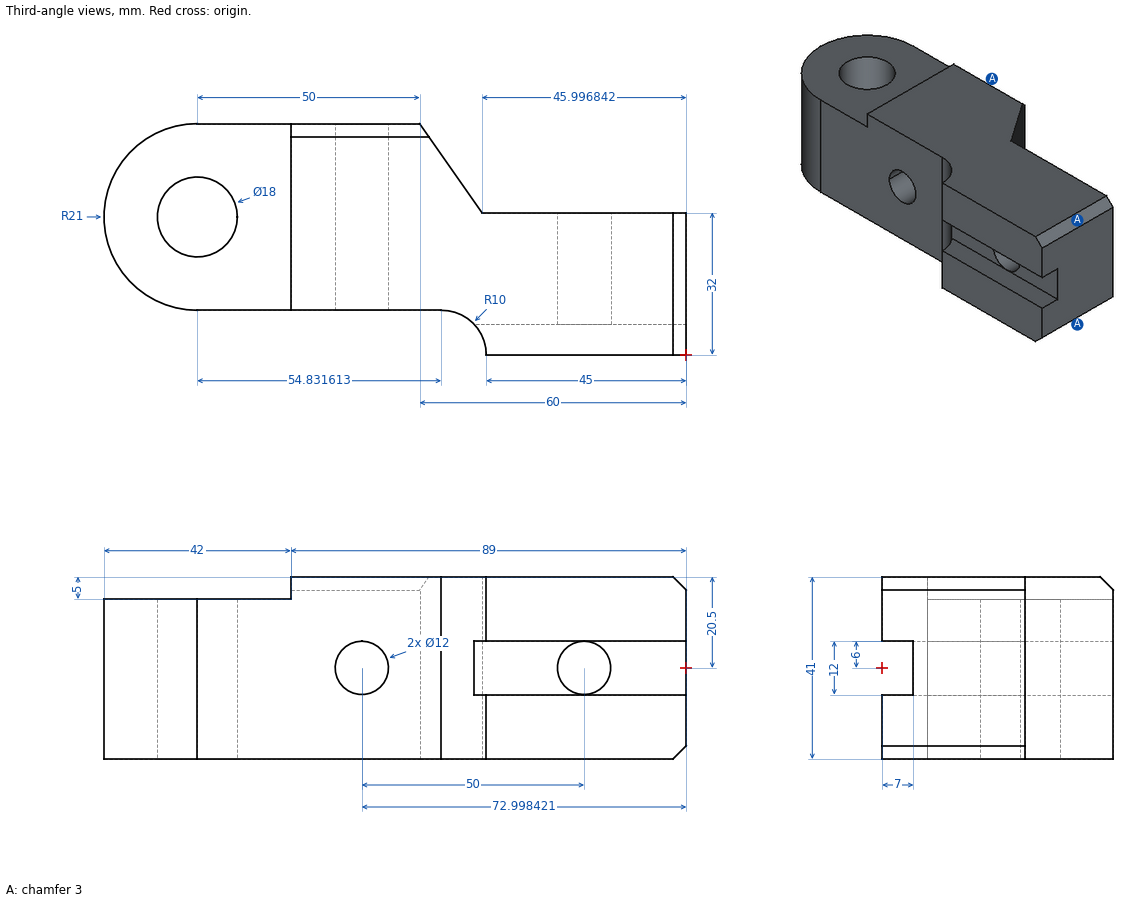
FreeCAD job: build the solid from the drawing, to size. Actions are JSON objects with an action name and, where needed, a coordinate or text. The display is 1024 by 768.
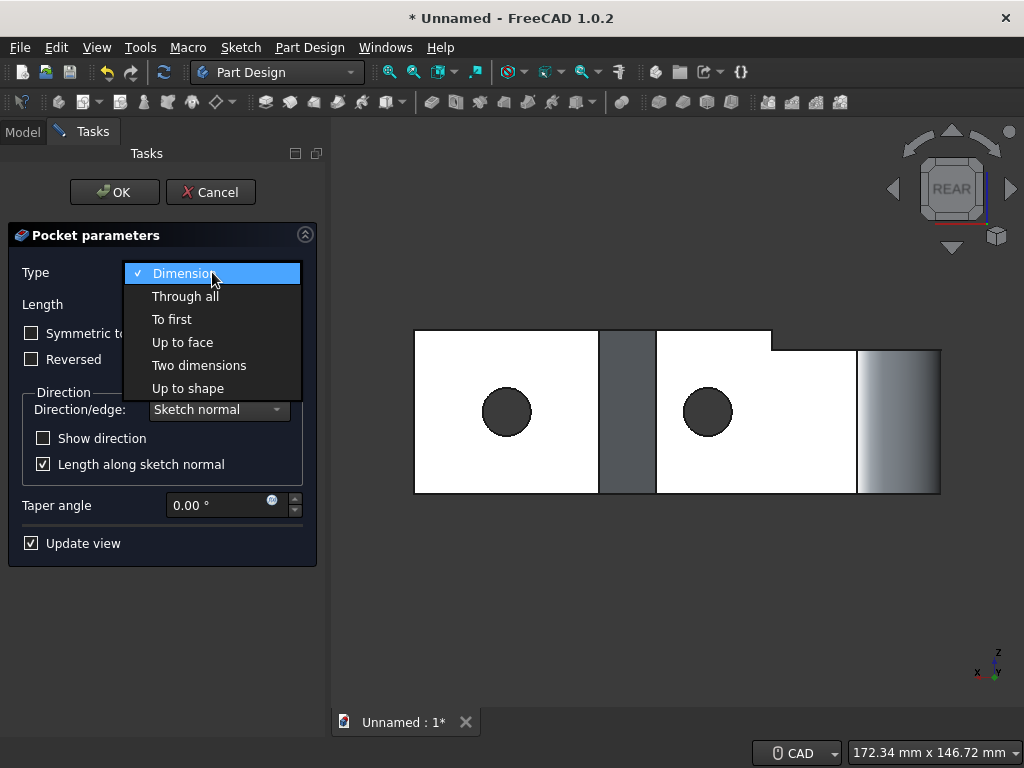
{"action": "left_click", "coordinate": [212, 296]}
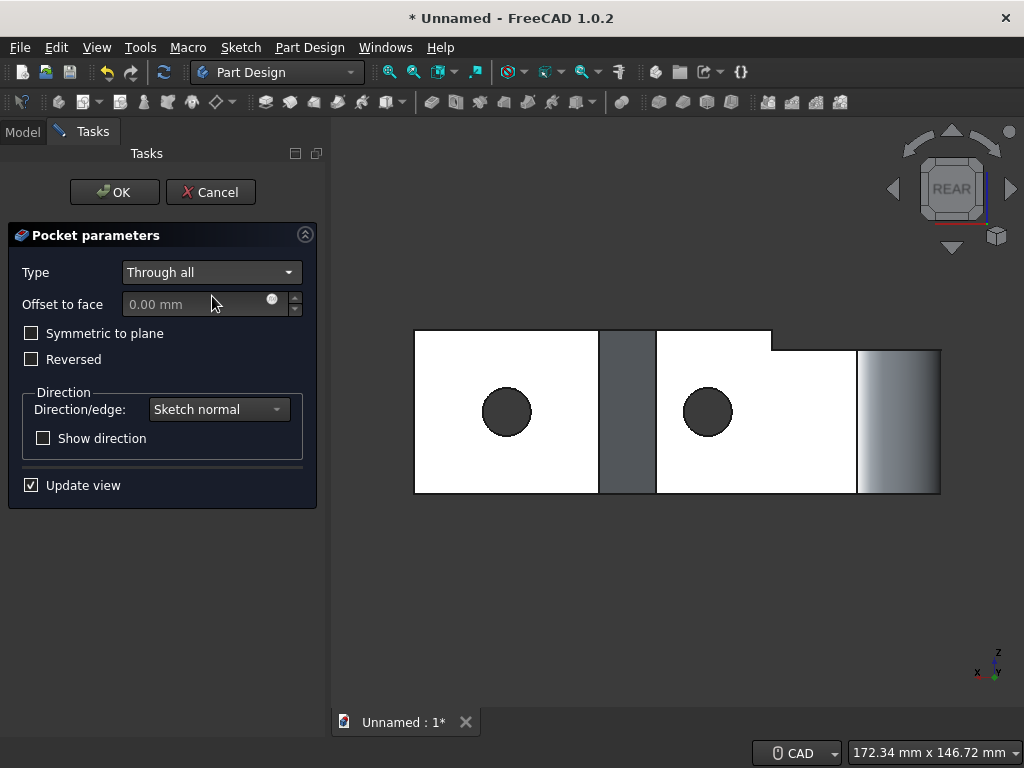
{"action": "left_click", "coordinate": [115, 192]}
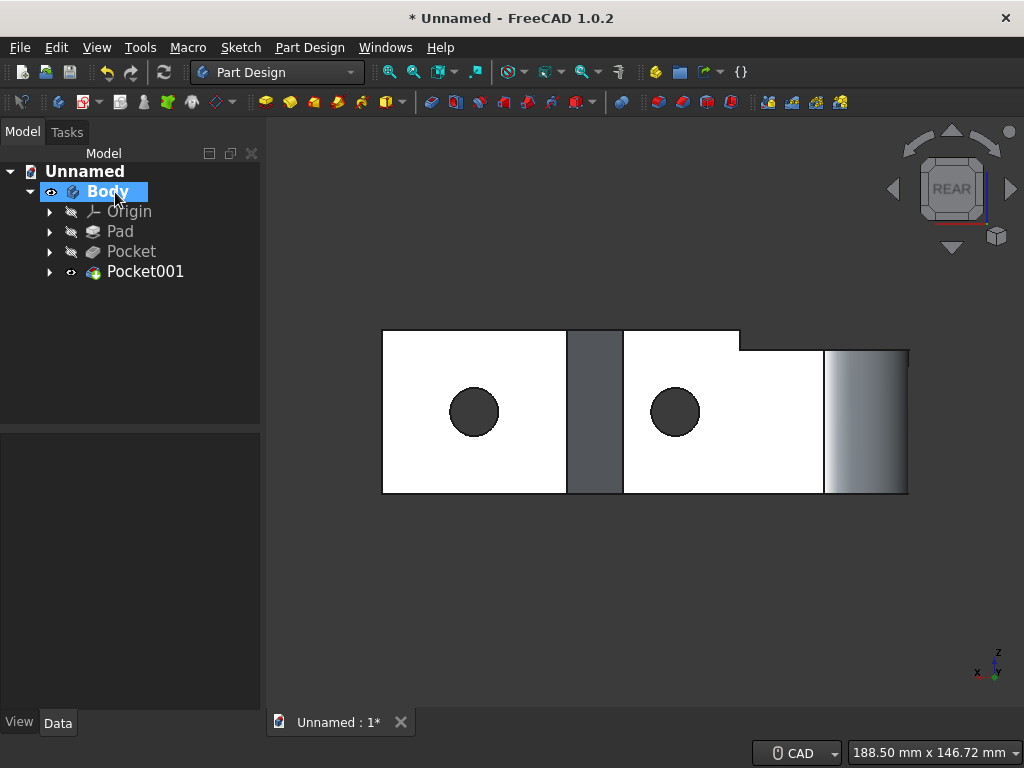
{"action": "left_click", "coordinate": [681, 329]}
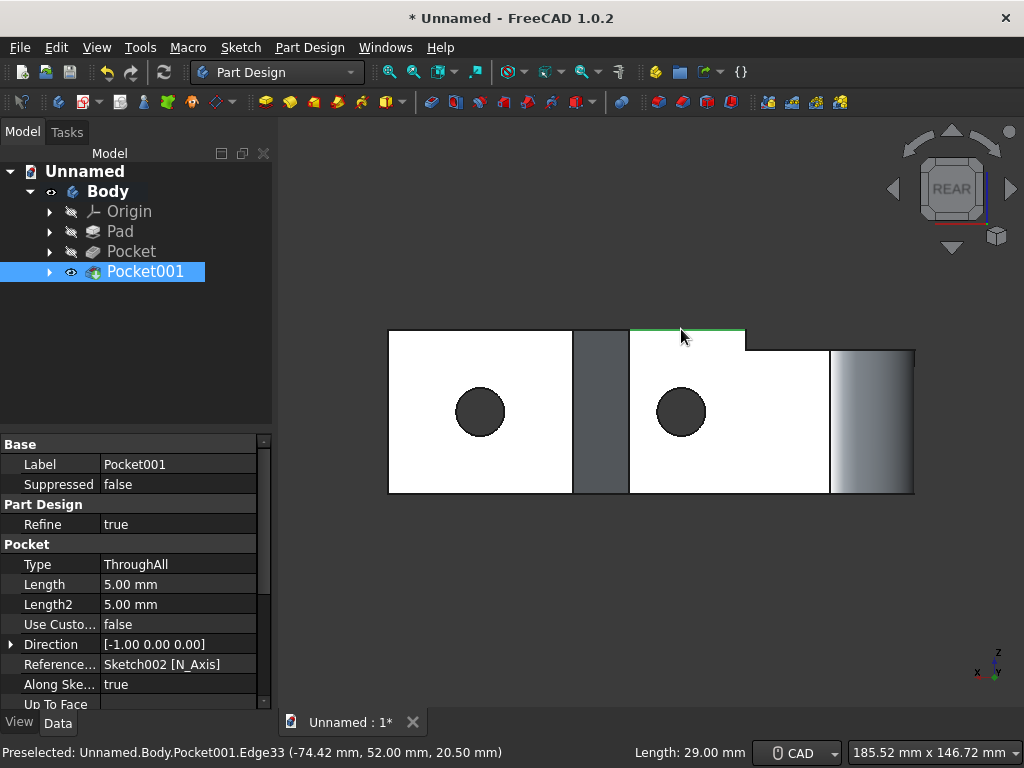
{"action": "key", "text": "0"}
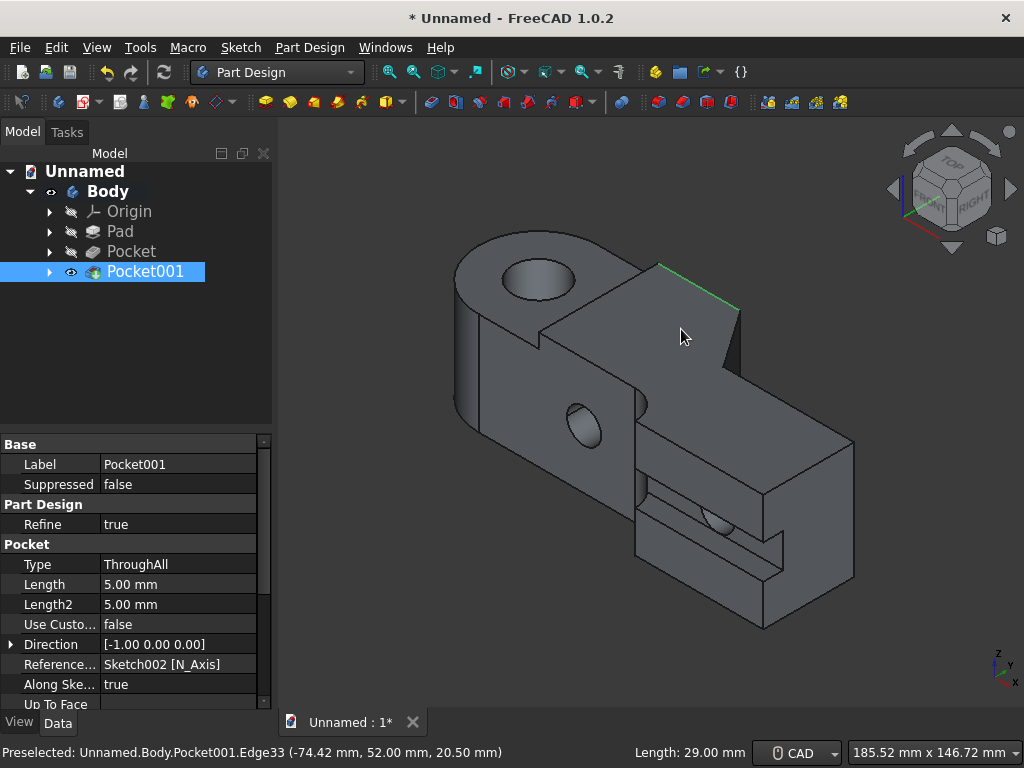
{"action": "left_click", "coordinate": [809, 468], "text": "ctrl"}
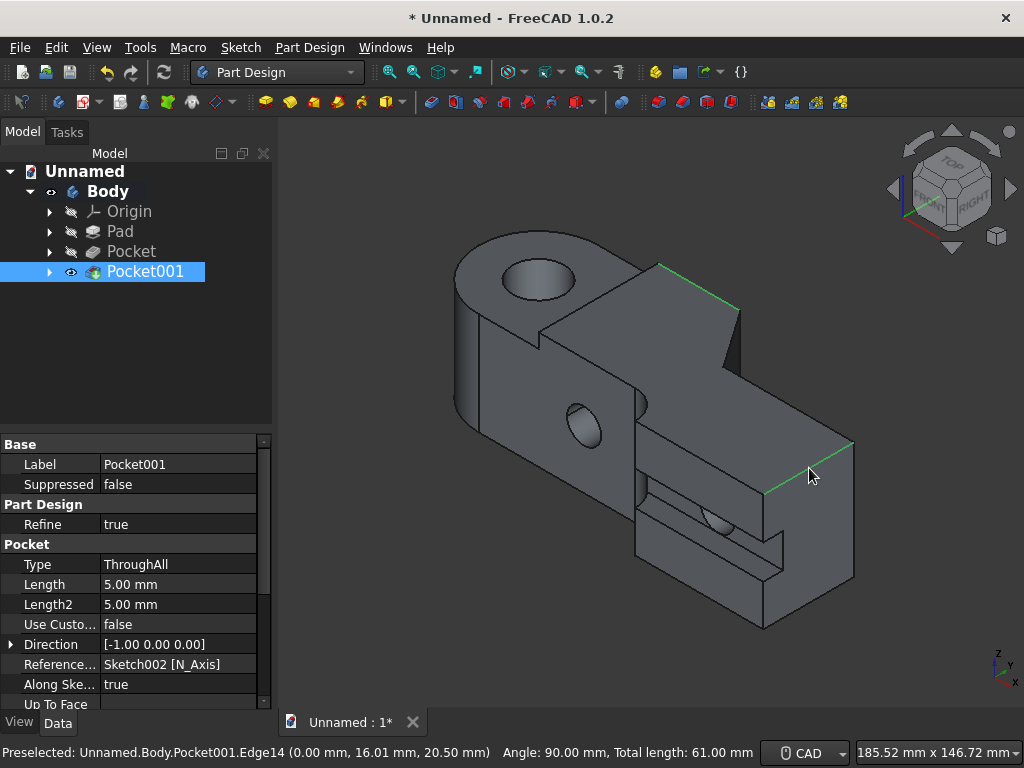
{"action": "key", "text": "2"}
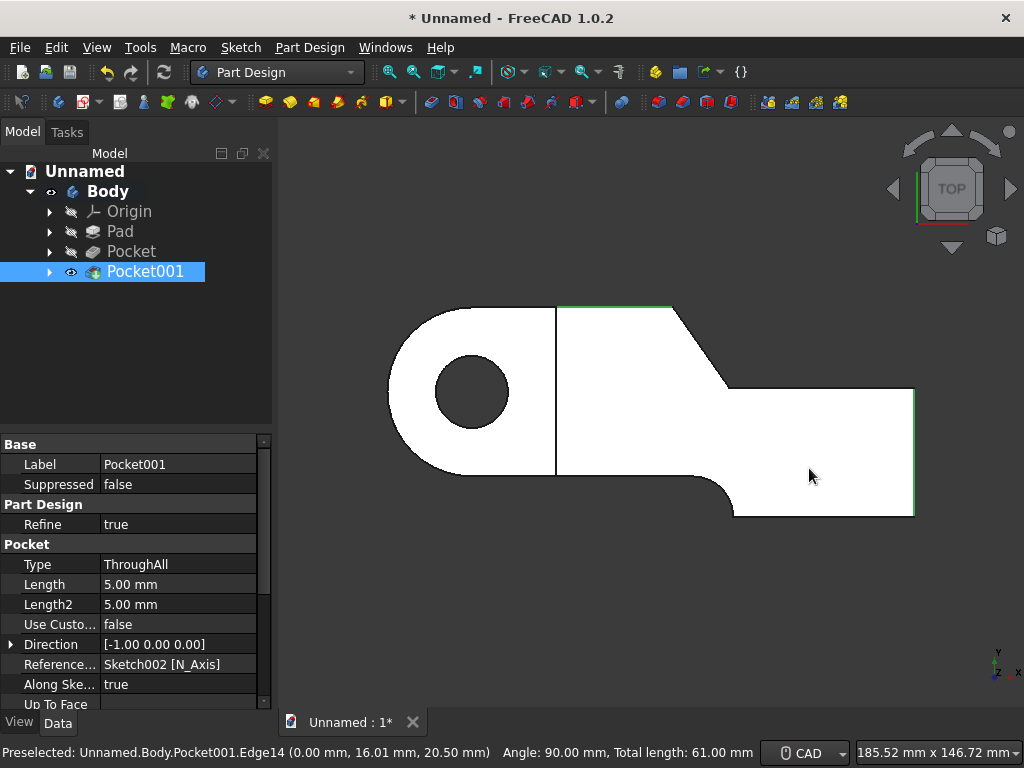
{"action": "key", "text": "1"}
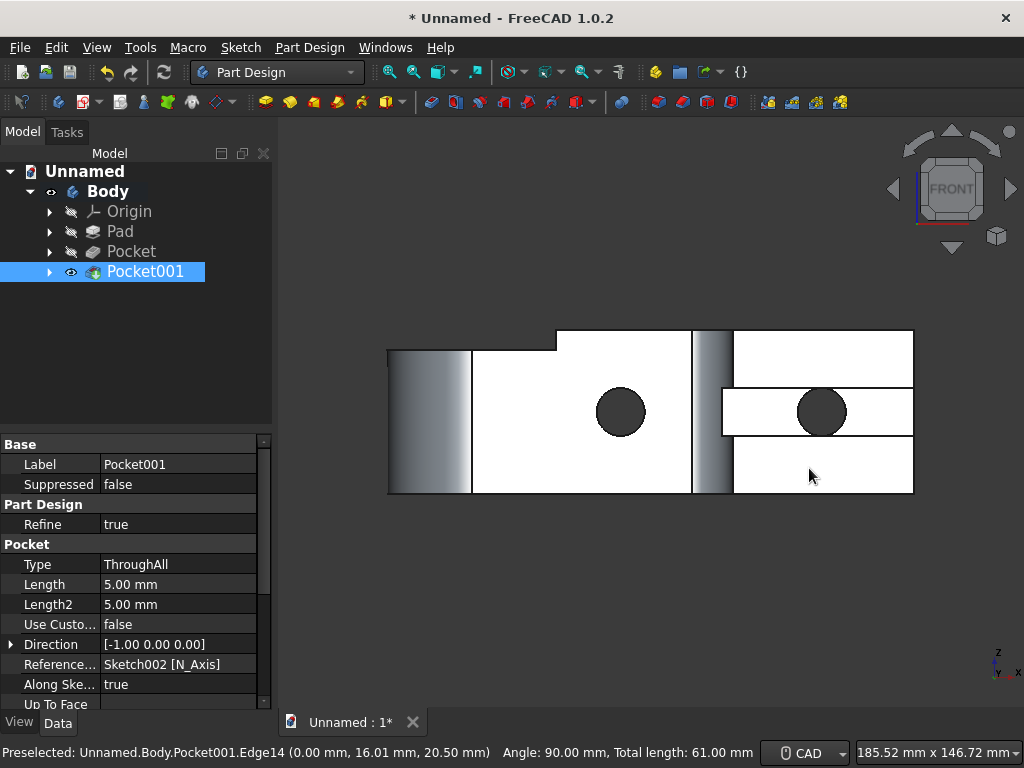
{"action": "key", "text": "3"}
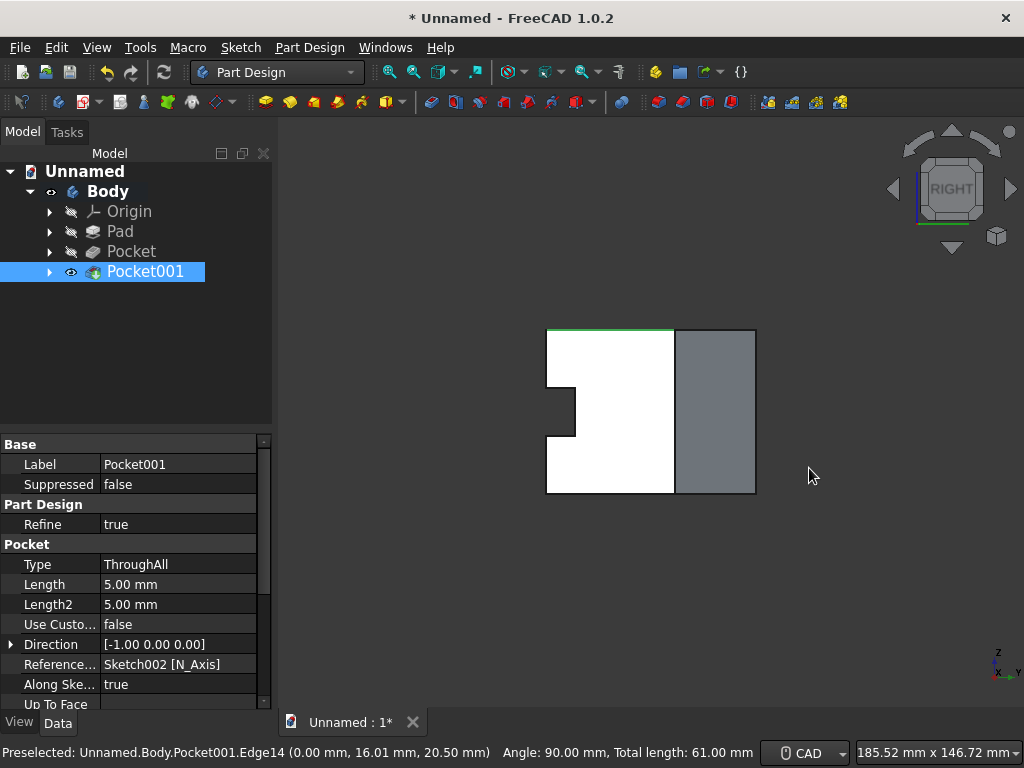
{"action": "left_click", "coordinate": [390, 72]}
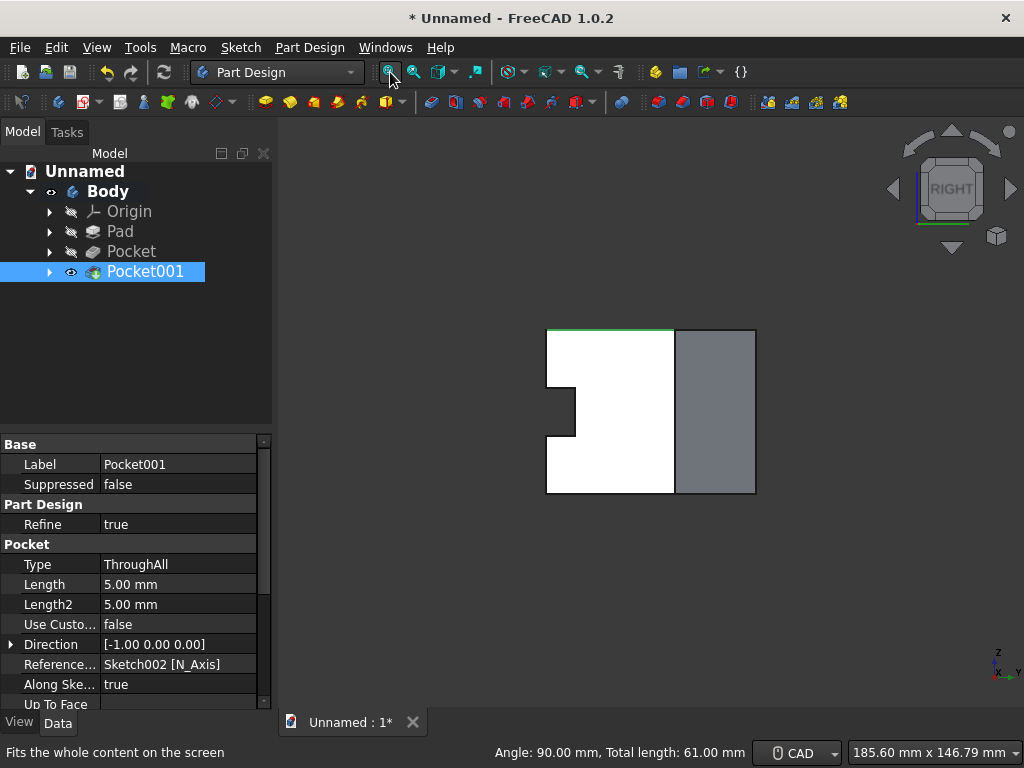
{"action": "left_click", "coordinate": [611, 493], "text": "ctrl"}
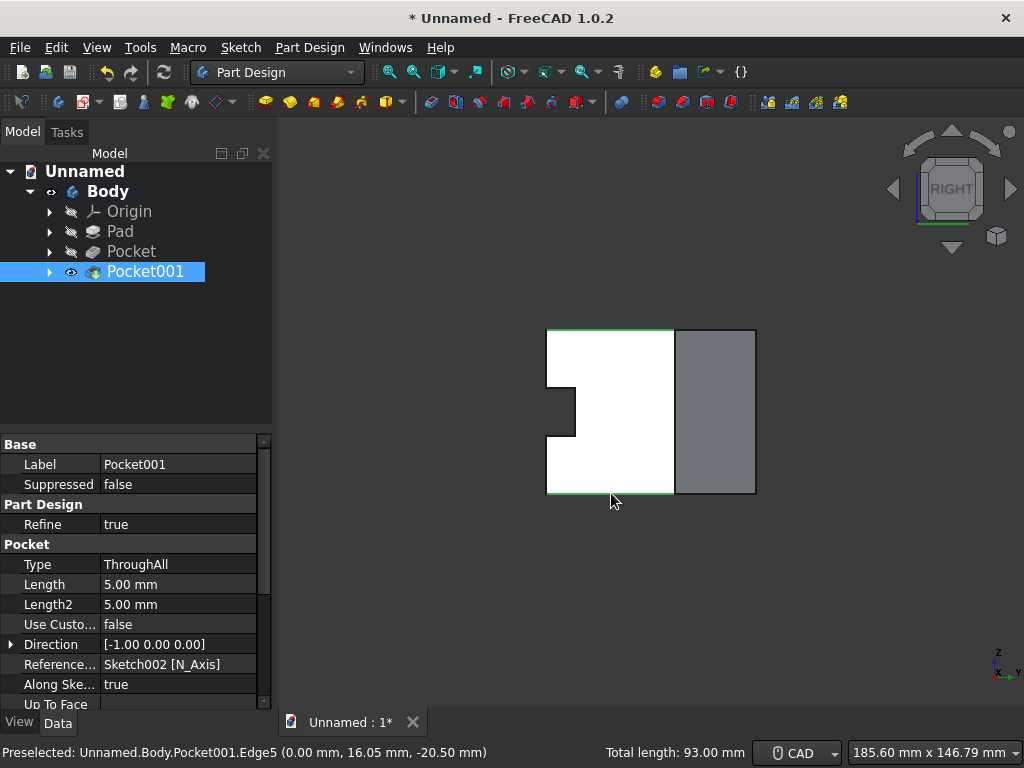
{"action": "left_click", "coordinate": [684, 102]}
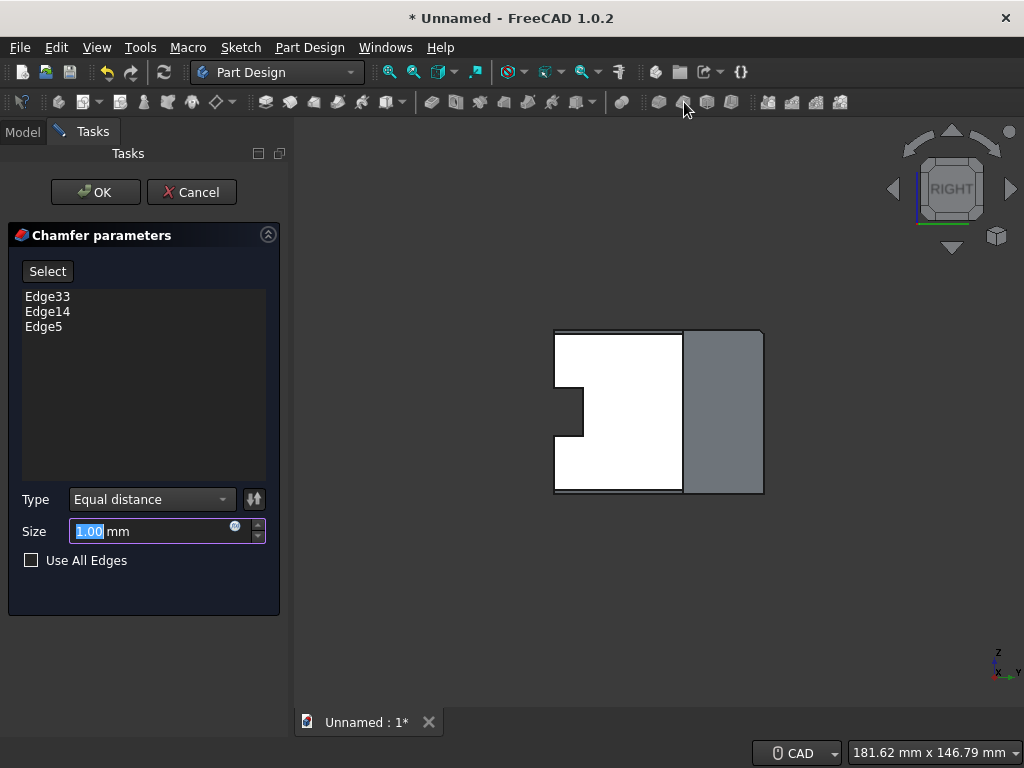
{"action": "type", "text": "3"}
{"action": "key", "text": "Tab"}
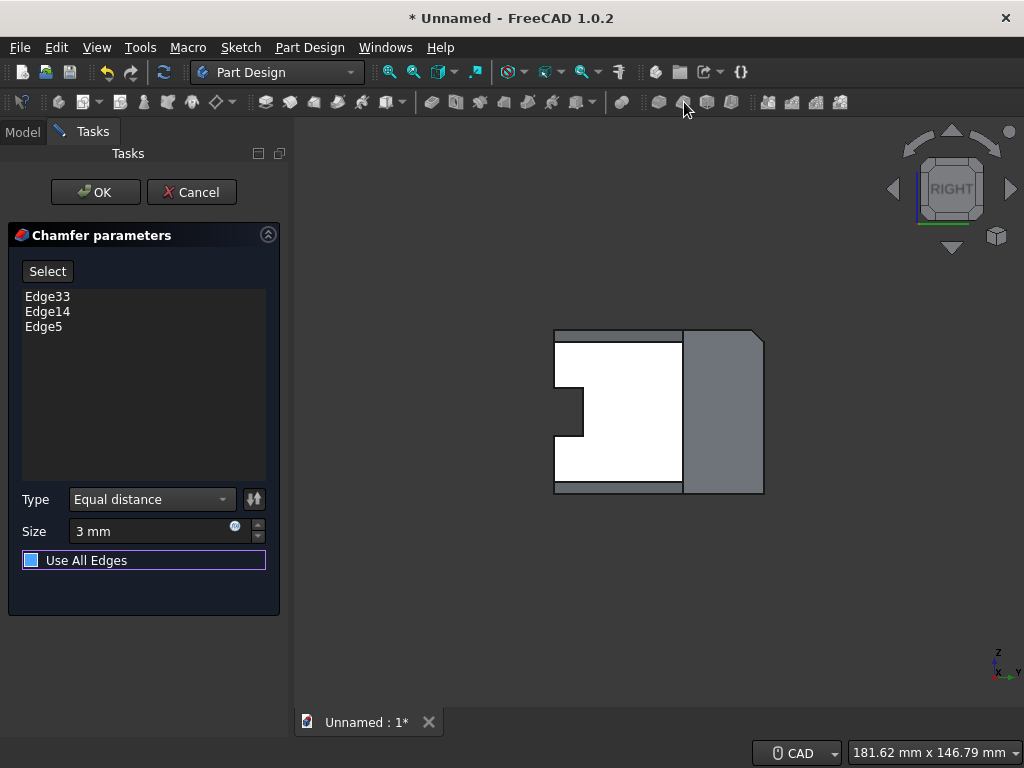
{"action": "left_click", "coordinate": [96, 192]}